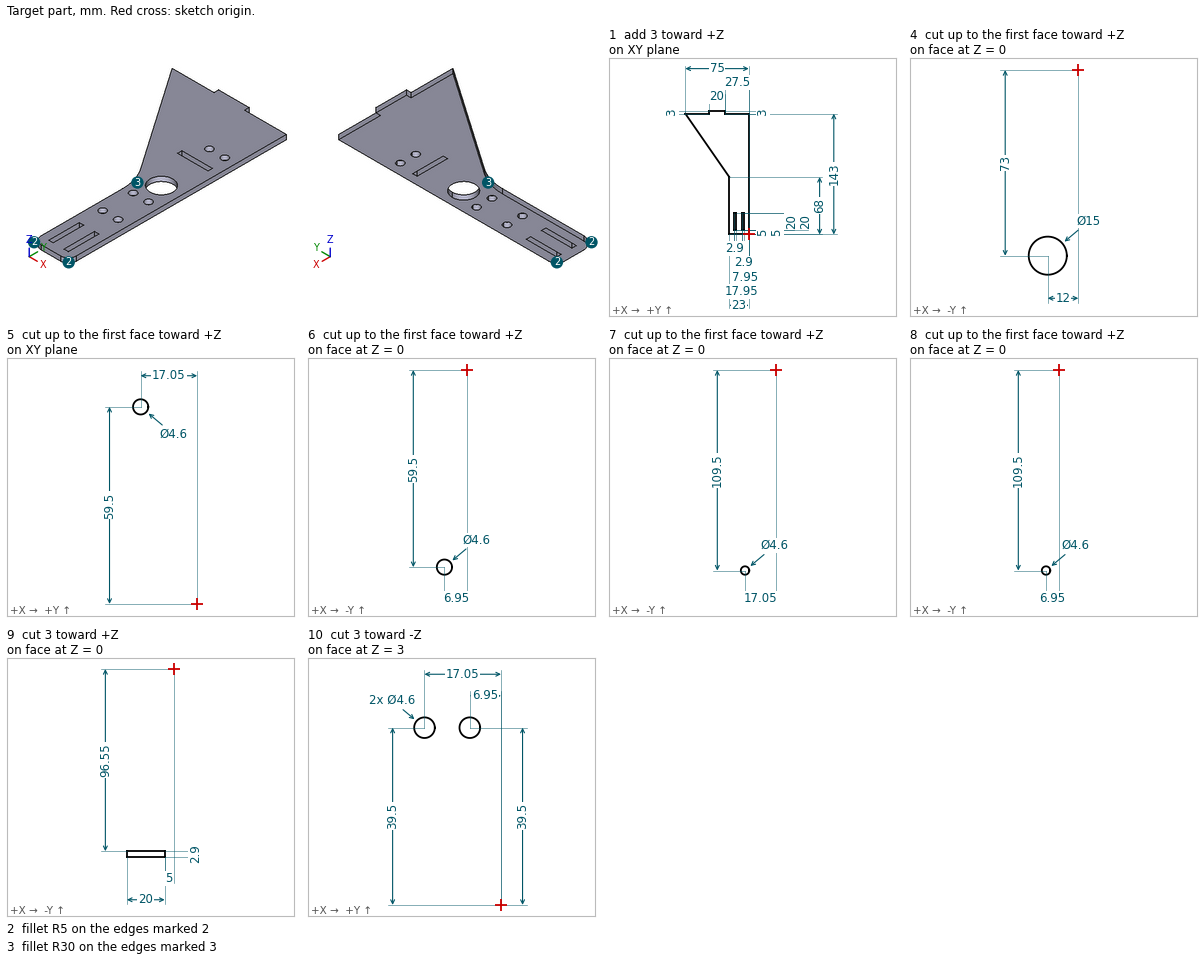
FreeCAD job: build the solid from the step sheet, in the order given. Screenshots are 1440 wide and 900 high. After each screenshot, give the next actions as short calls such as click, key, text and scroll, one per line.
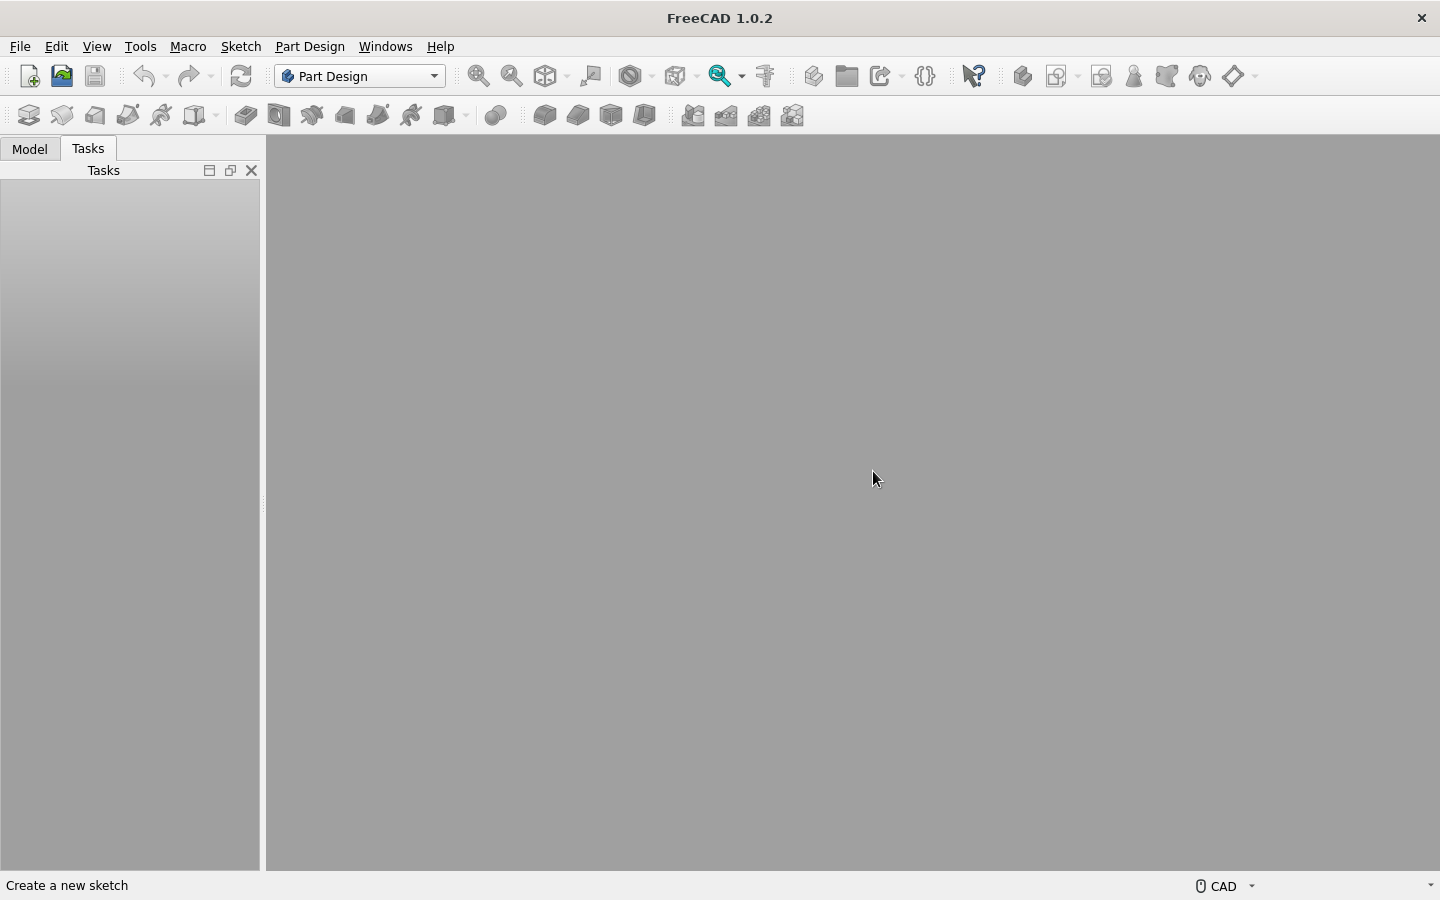
click(29, 76)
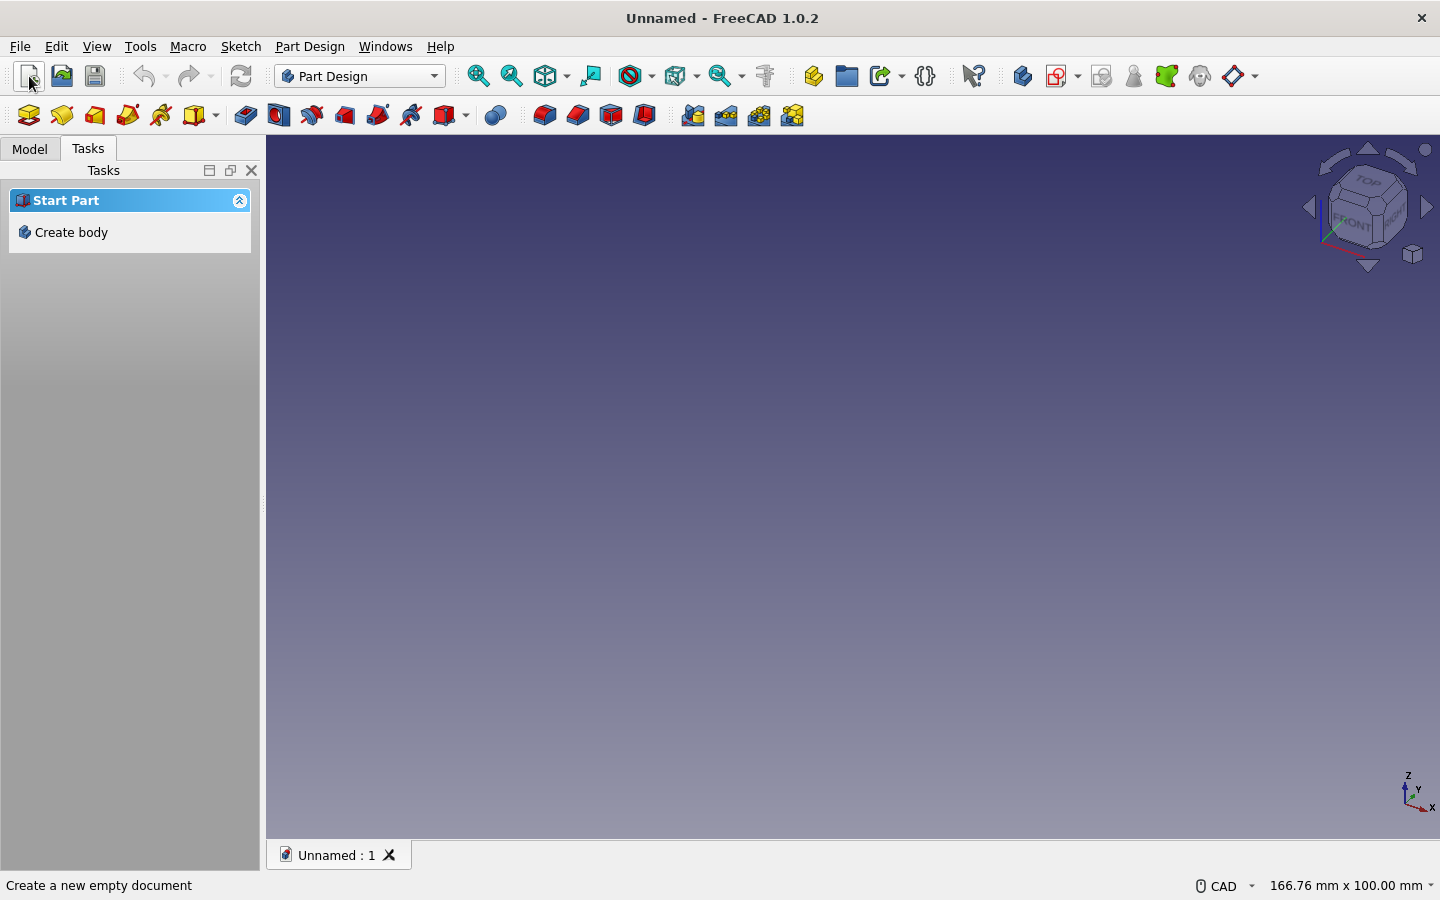
click(1056, 76)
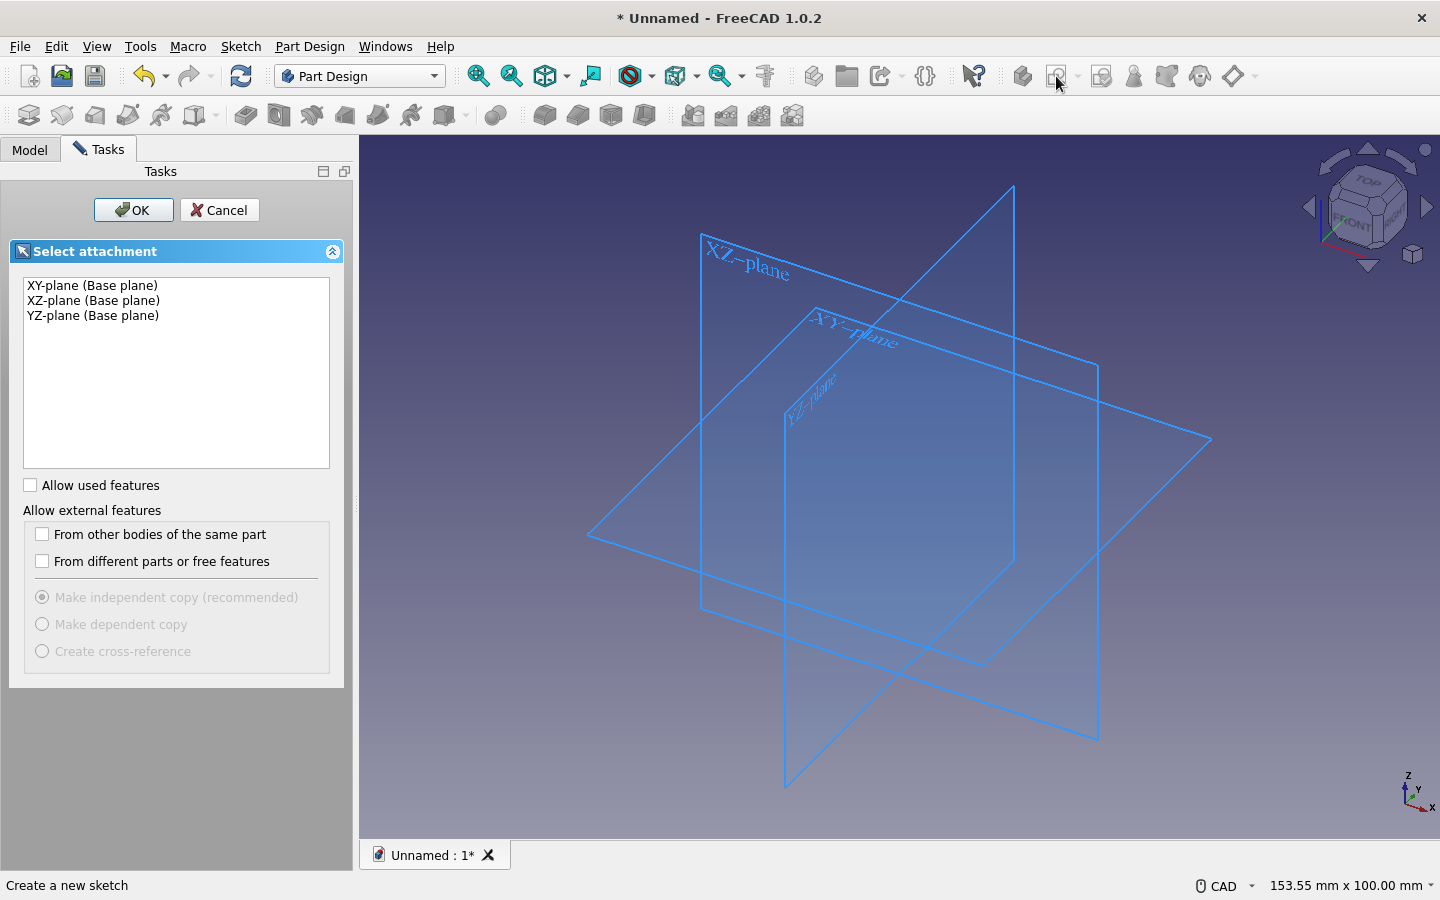
click(84, 286)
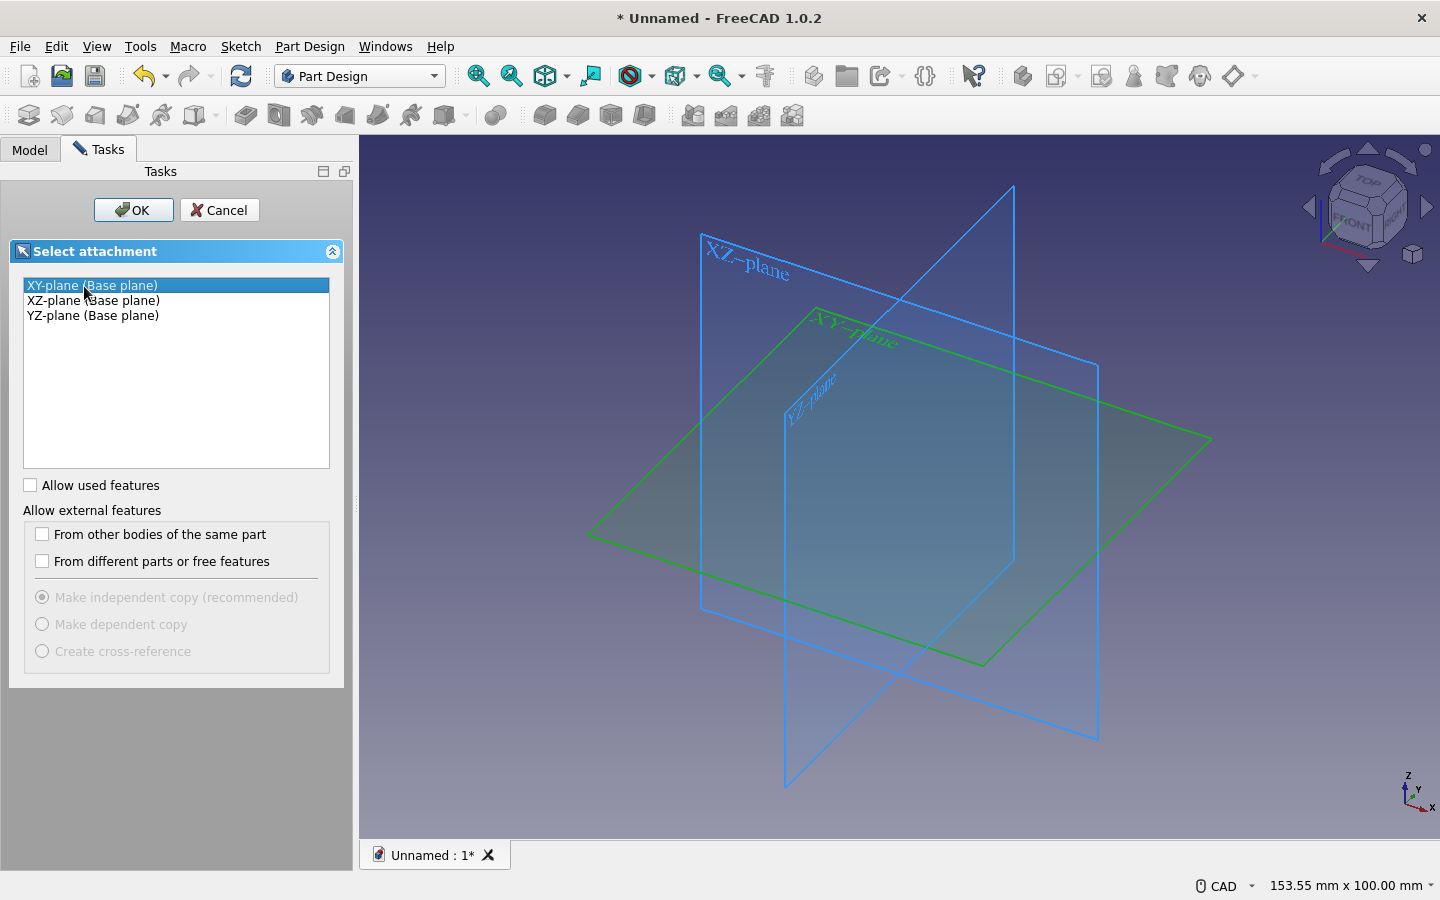
click(134, 210)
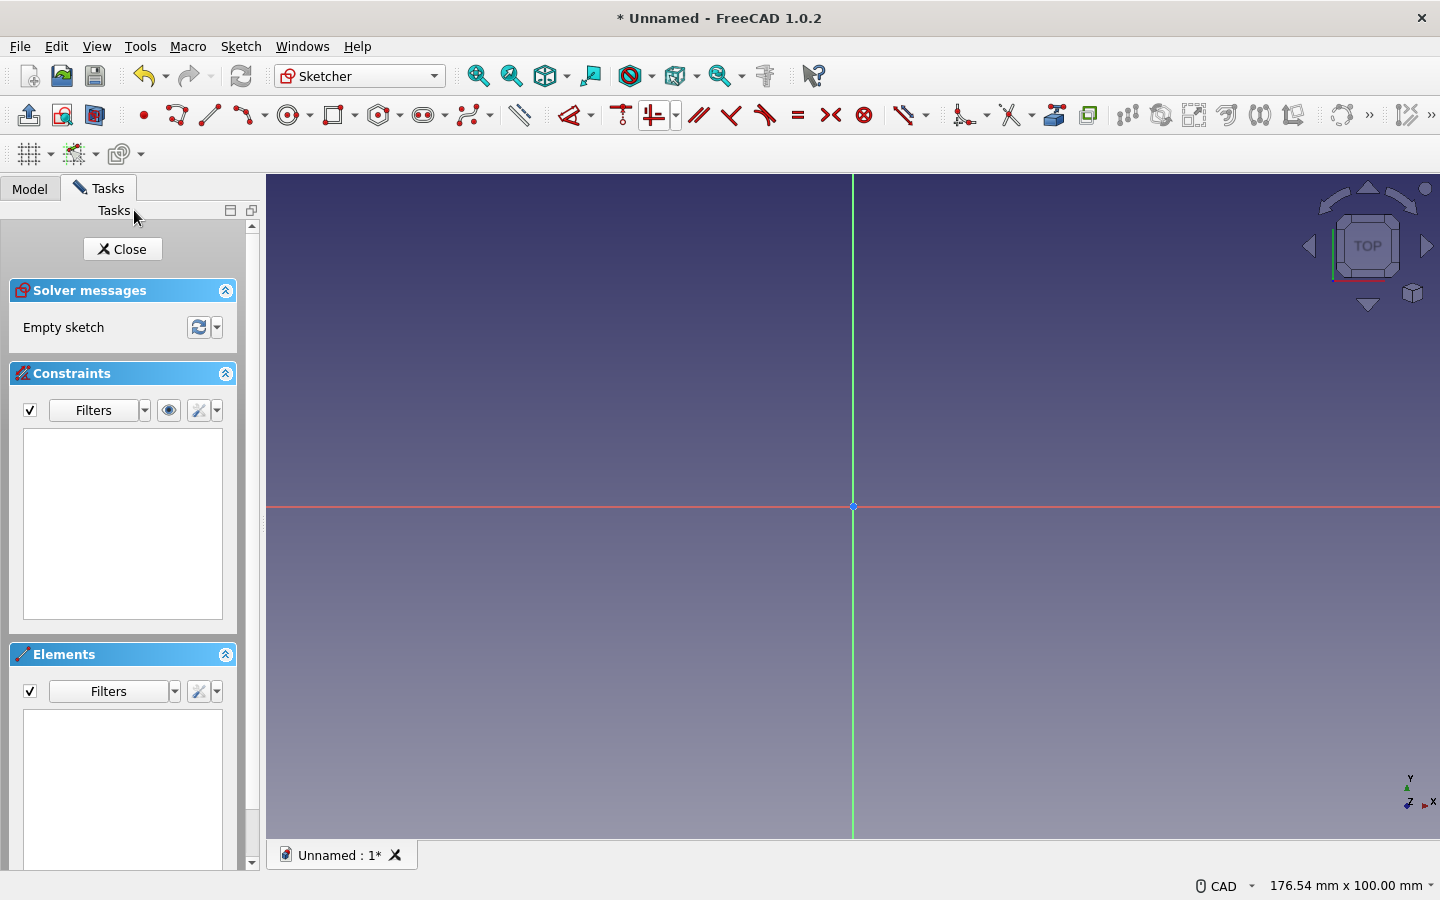
scroll(932, 811, down, 4)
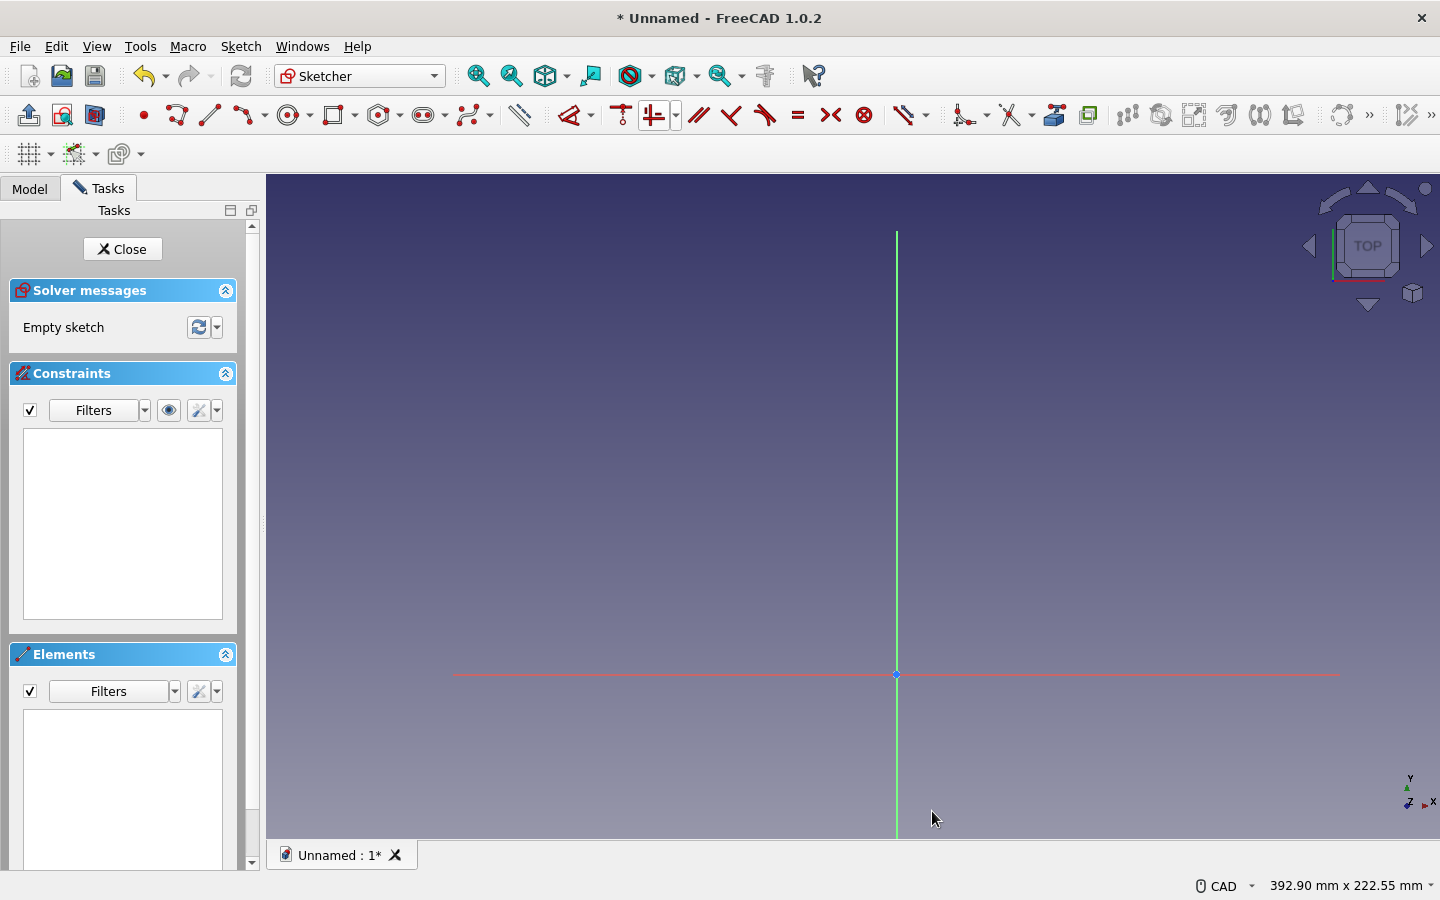
key(g)
key(m)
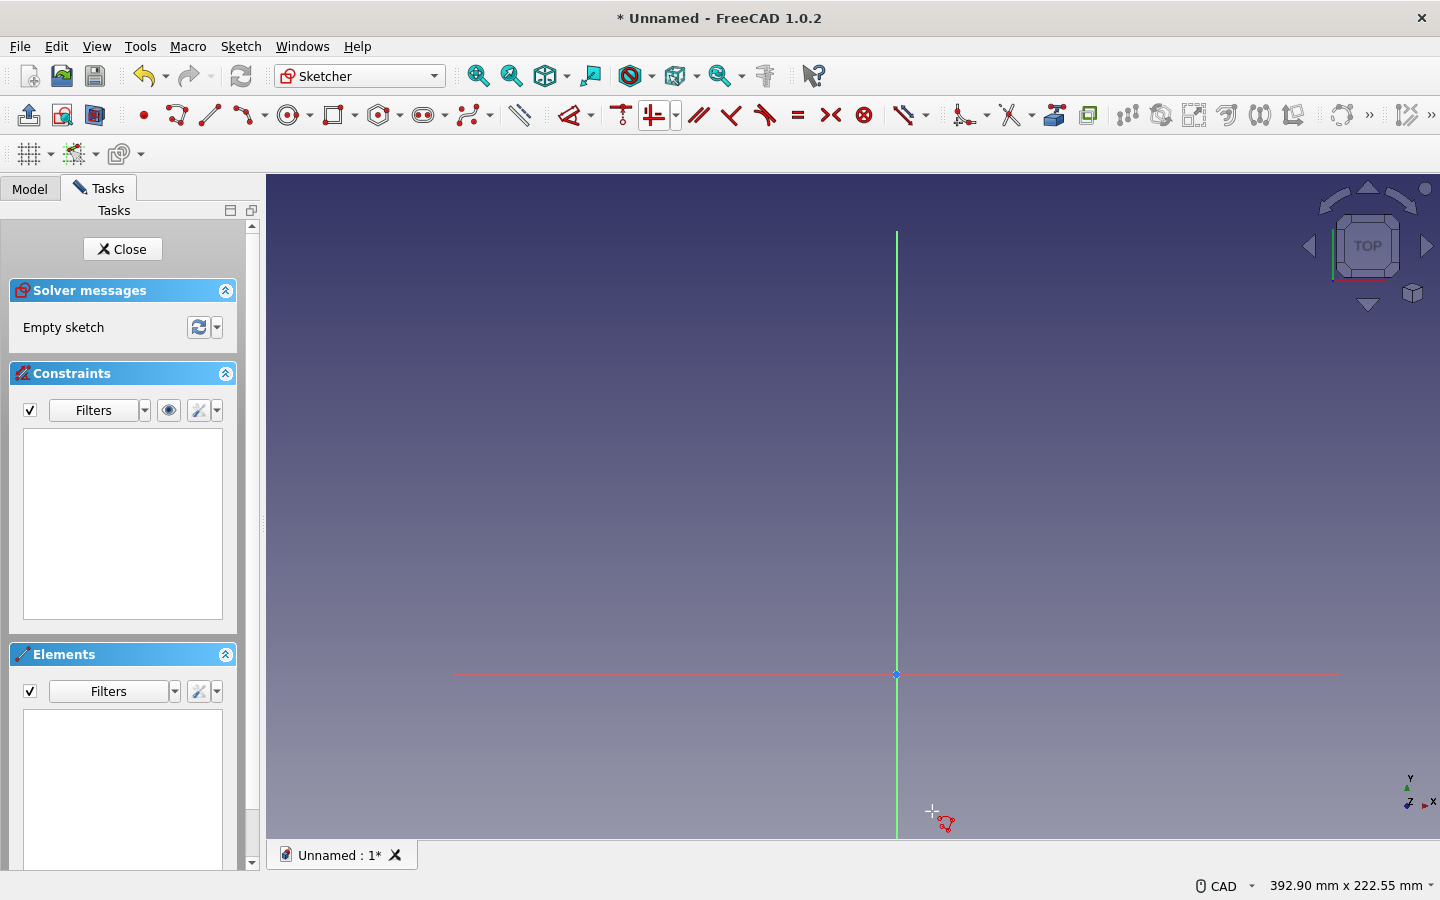
click(897, 675)
click(888, 247)
click(815, 247)